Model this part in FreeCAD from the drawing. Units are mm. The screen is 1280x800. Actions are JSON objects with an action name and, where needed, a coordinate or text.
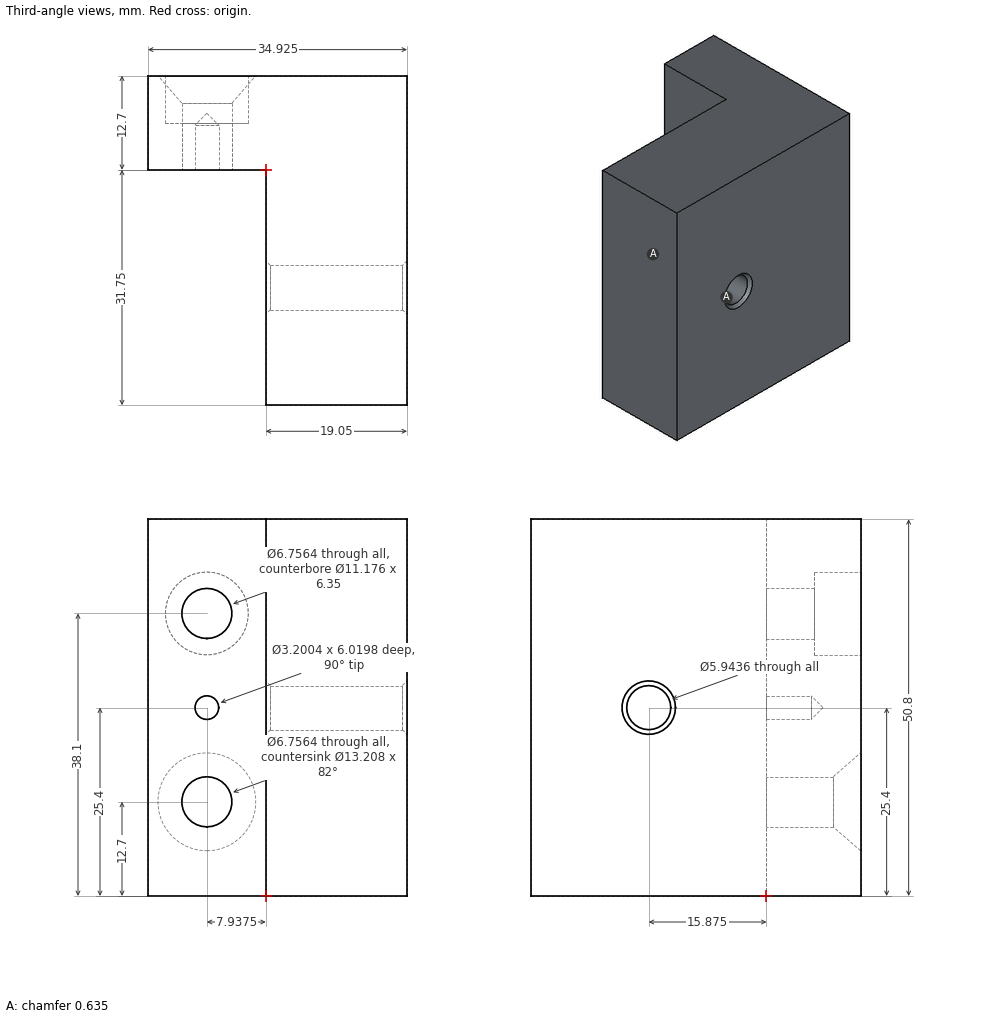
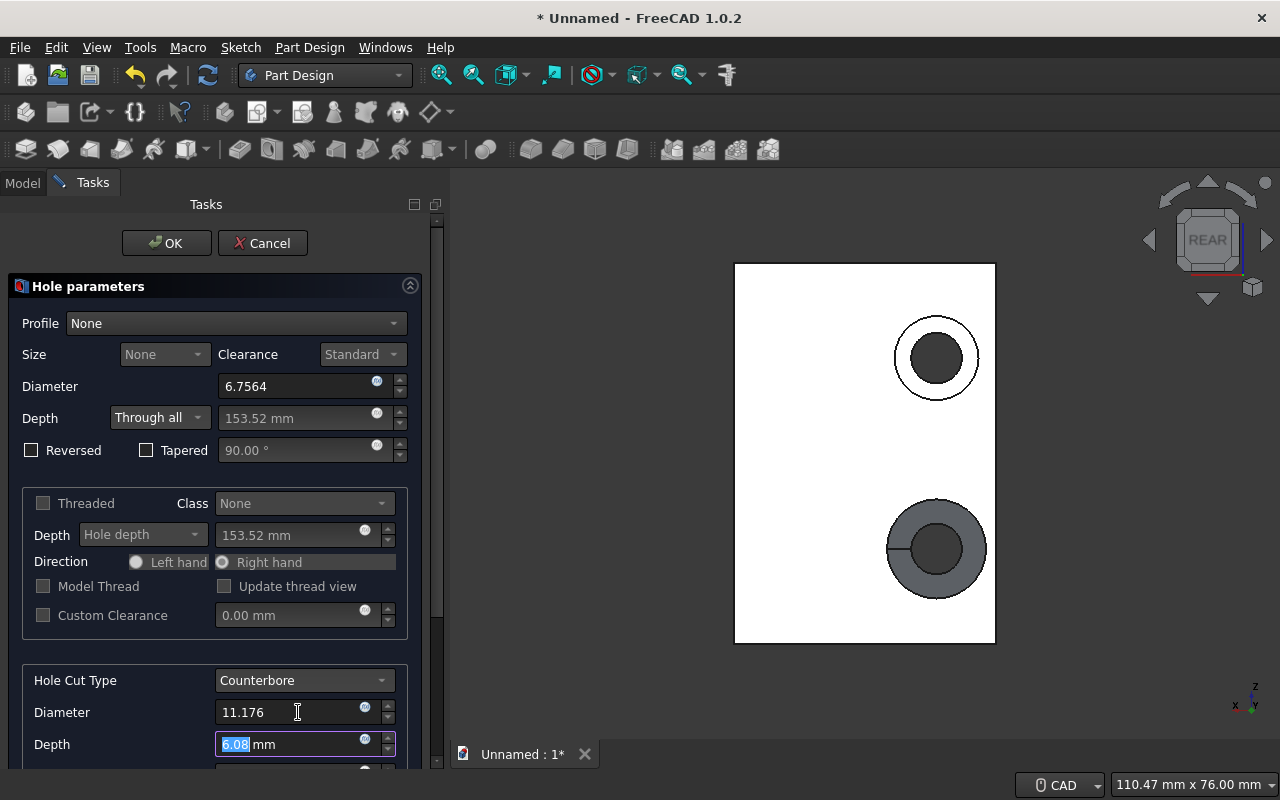
{"action": "type", "text": "6.35"}
{"action": "key", "text": "Tab"}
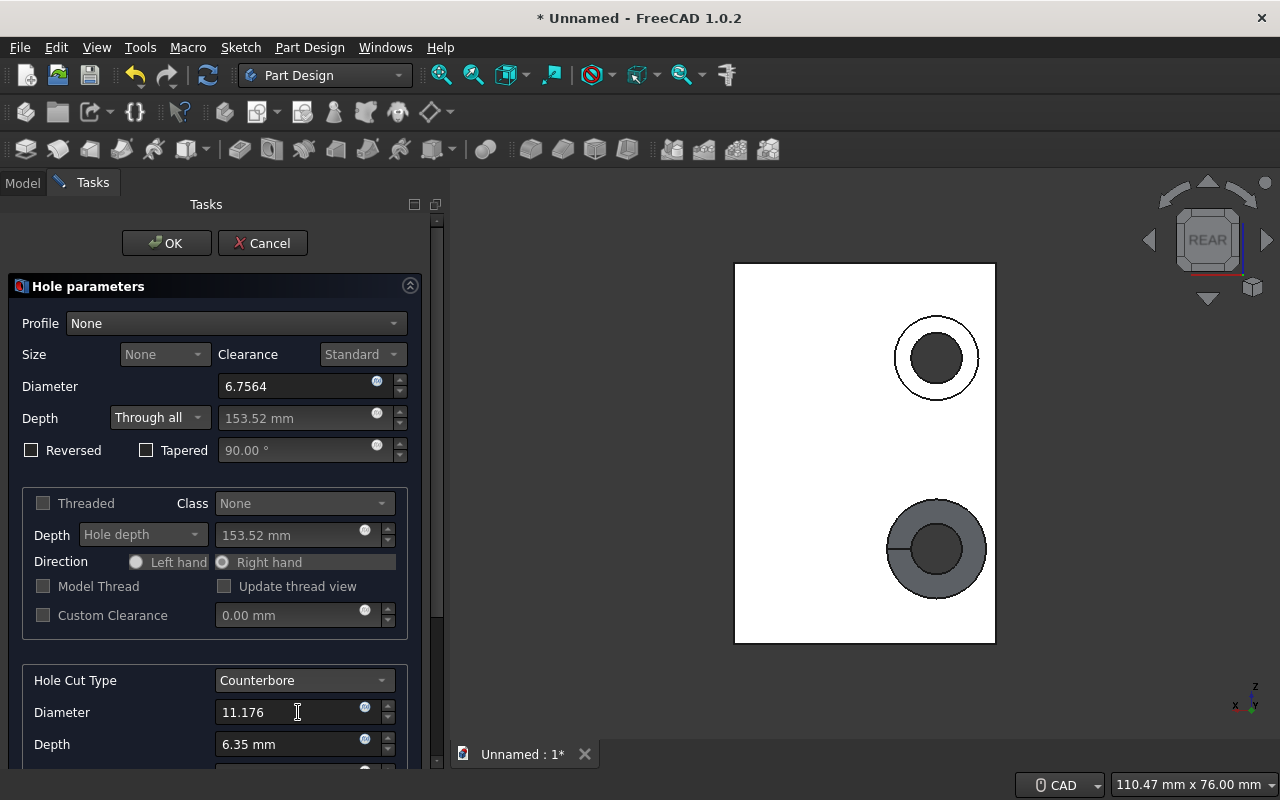
{"action": "left_click", "coordinate": [167, 243]}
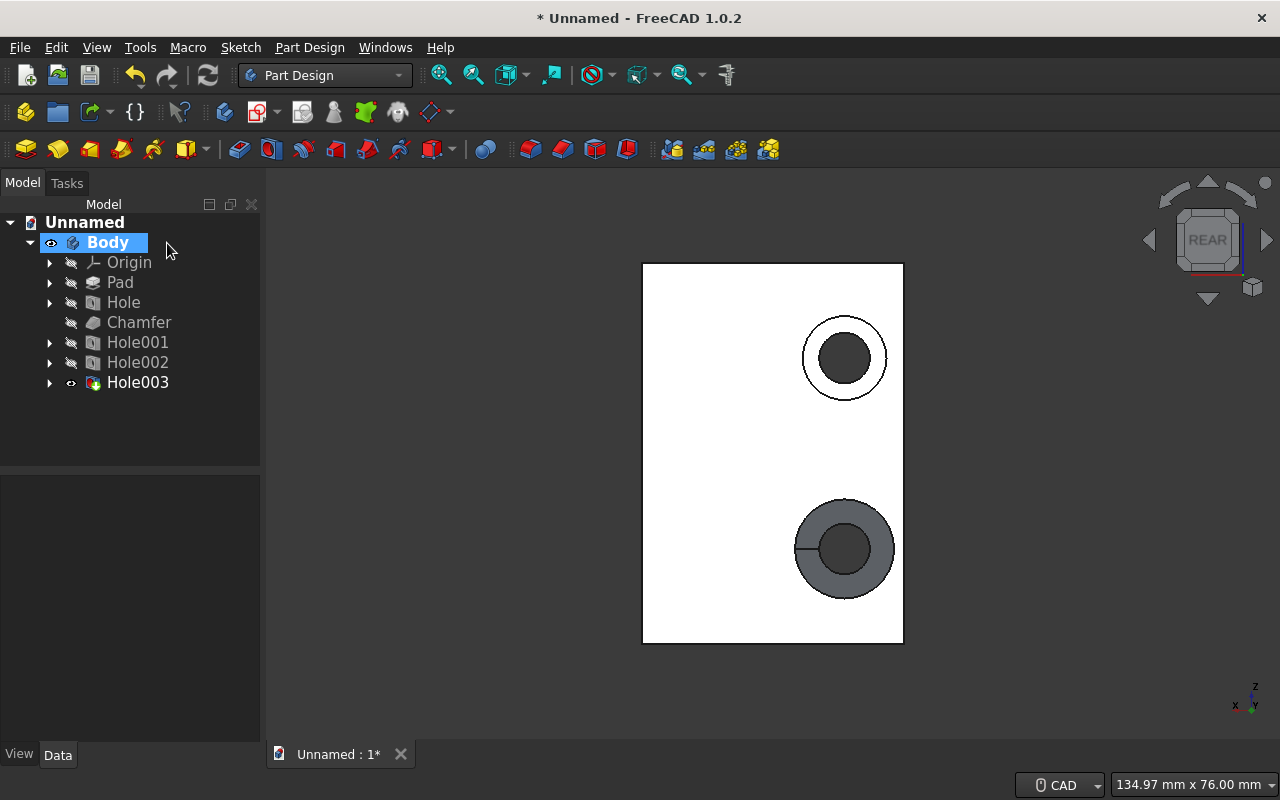
{"action": "key", "text": "0"}